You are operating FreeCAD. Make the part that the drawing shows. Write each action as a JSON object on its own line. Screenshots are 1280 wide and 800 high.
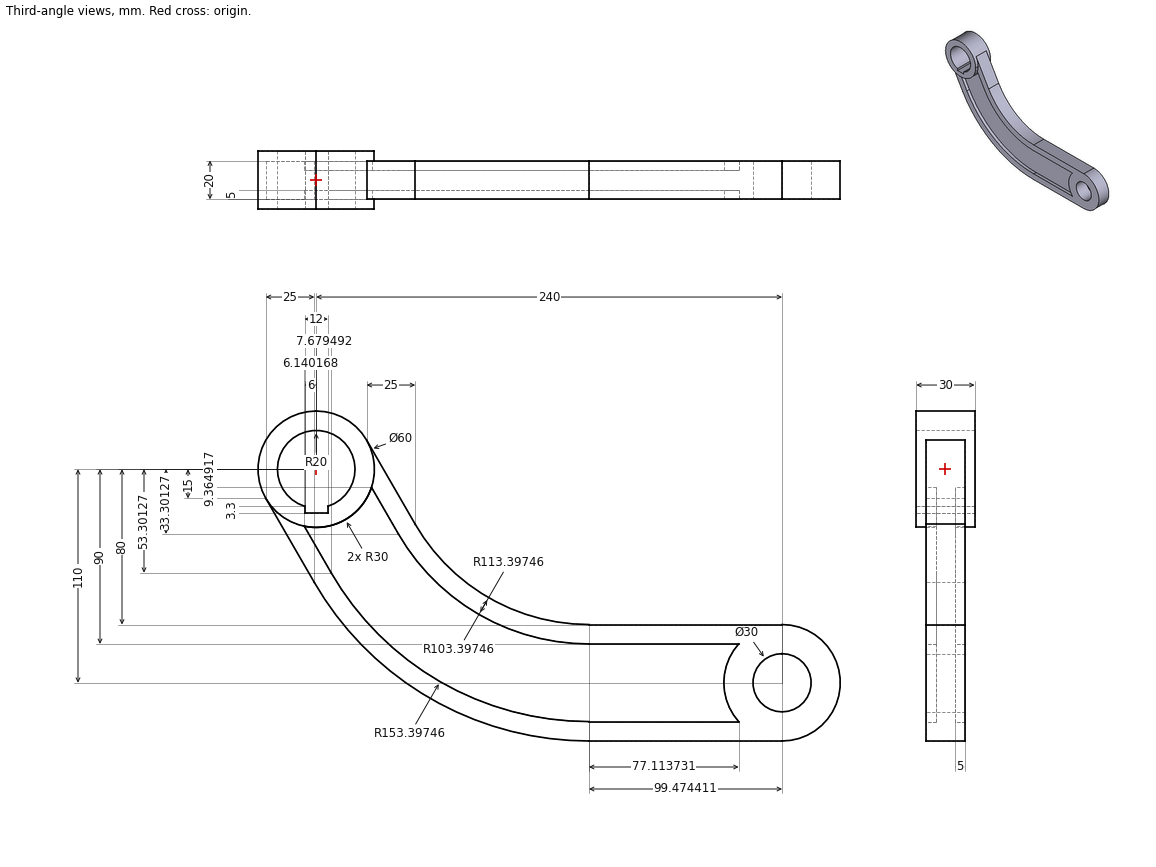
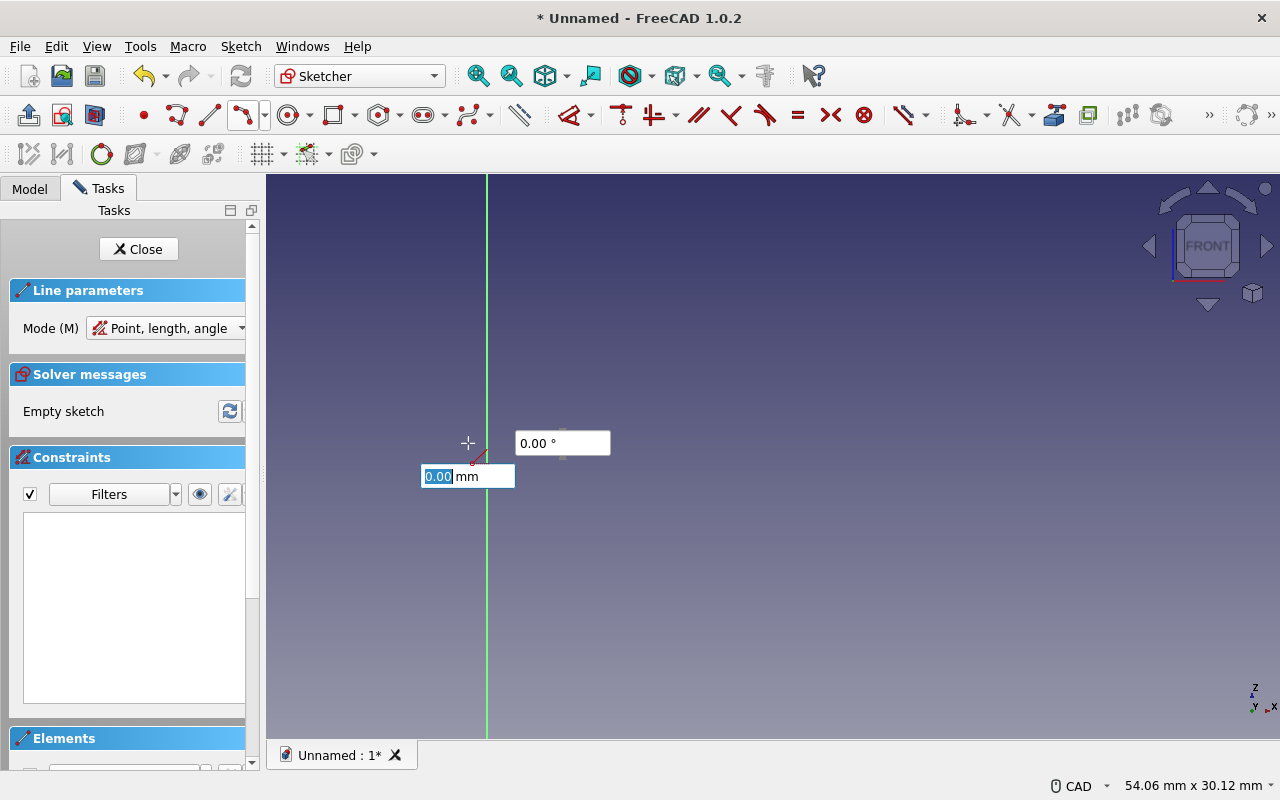
{"action": "scroll", "coordinate": [446, 448], "scroll_direction": "down", "scroll_amount": 11}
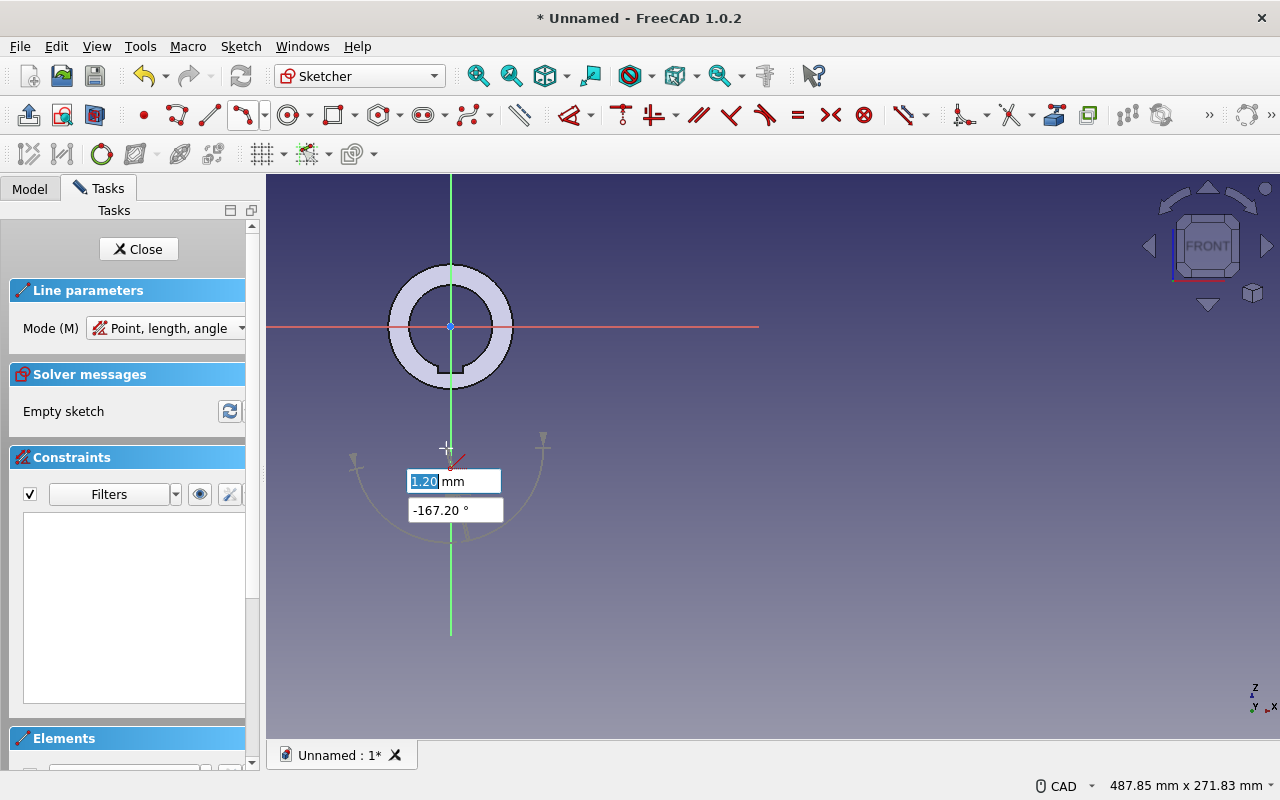
{"action": "left_click", "coordinate": [397, 358]}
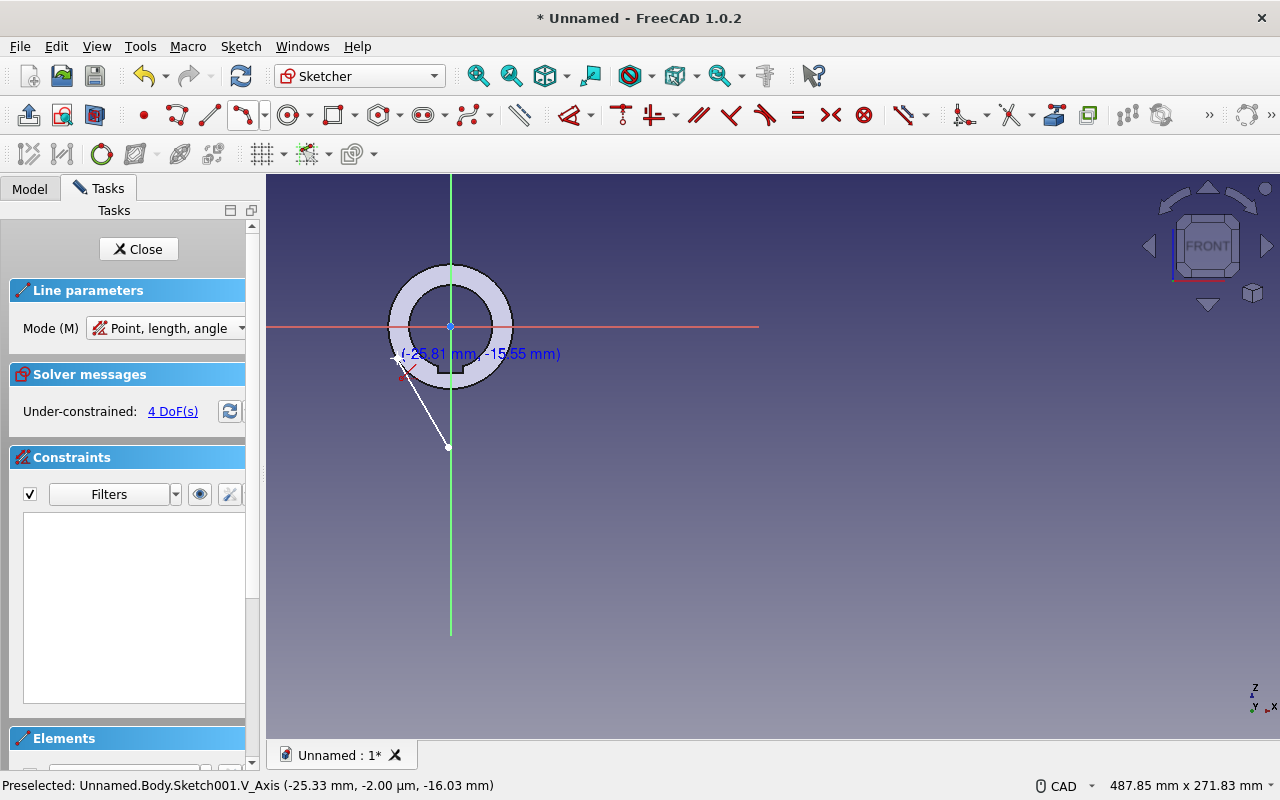
{"action": "left_click", "coordinate": [505, 296]}
{"action": "left_click", "coordinate": [557, 386]}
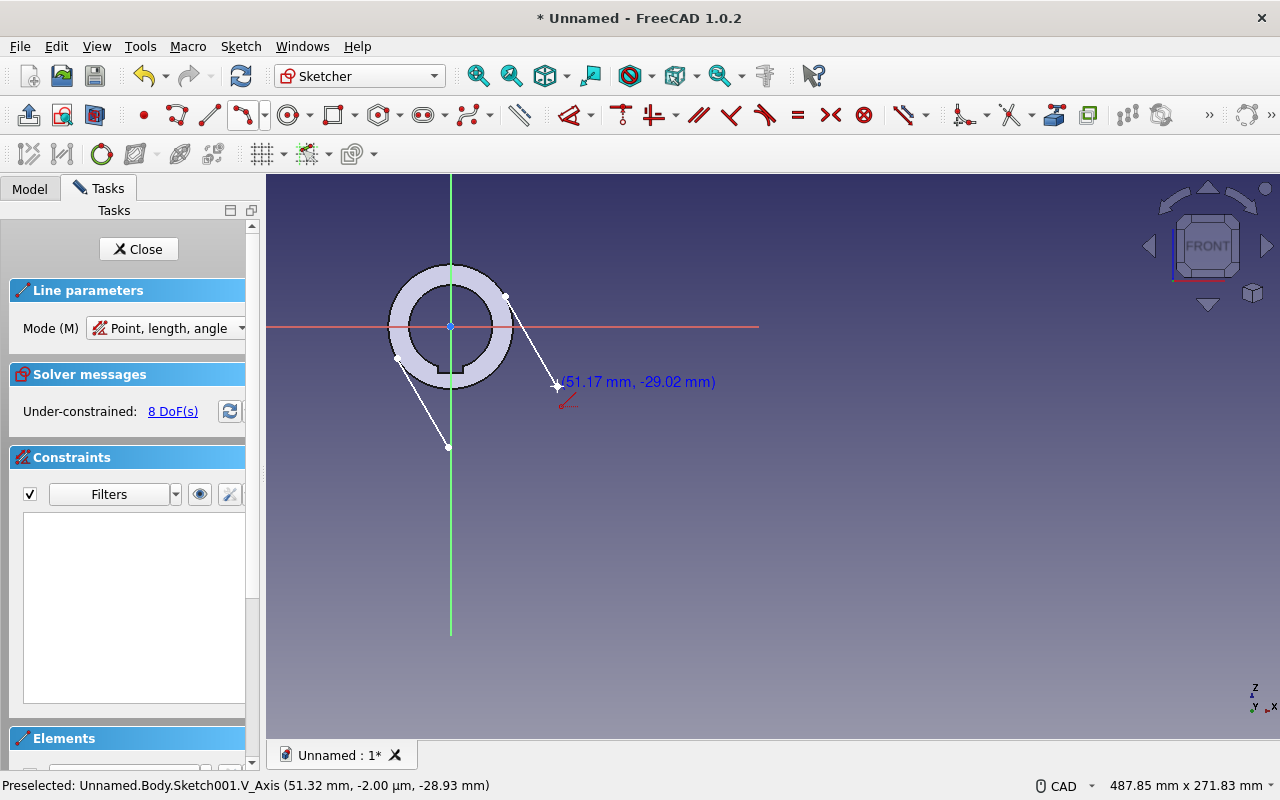
{"action": "left_click", "coordinate": [743, 493]}
{"action": "left_click", "coordinate": [949, 493]}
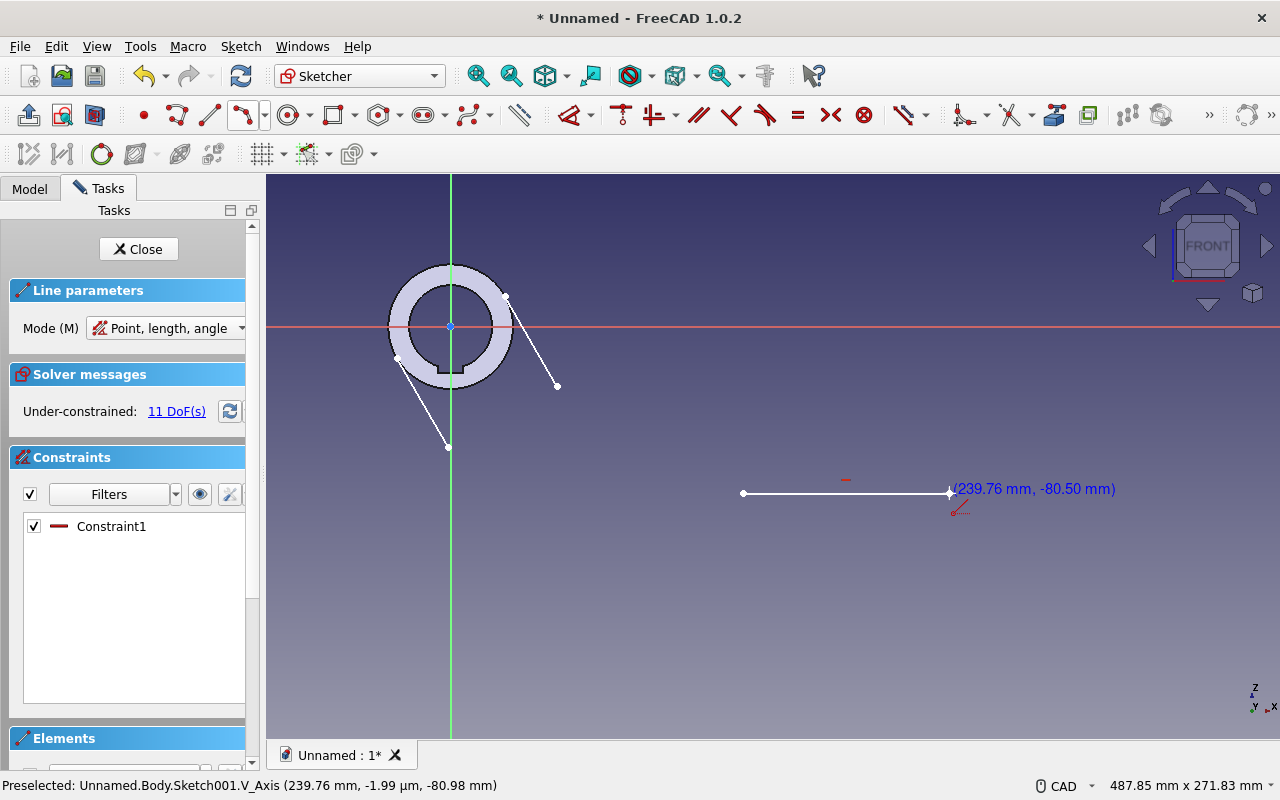
{"action": "left_click", "coordinate": [949, 618]}
{"action": "left_click", "coordinate": [743, 618]}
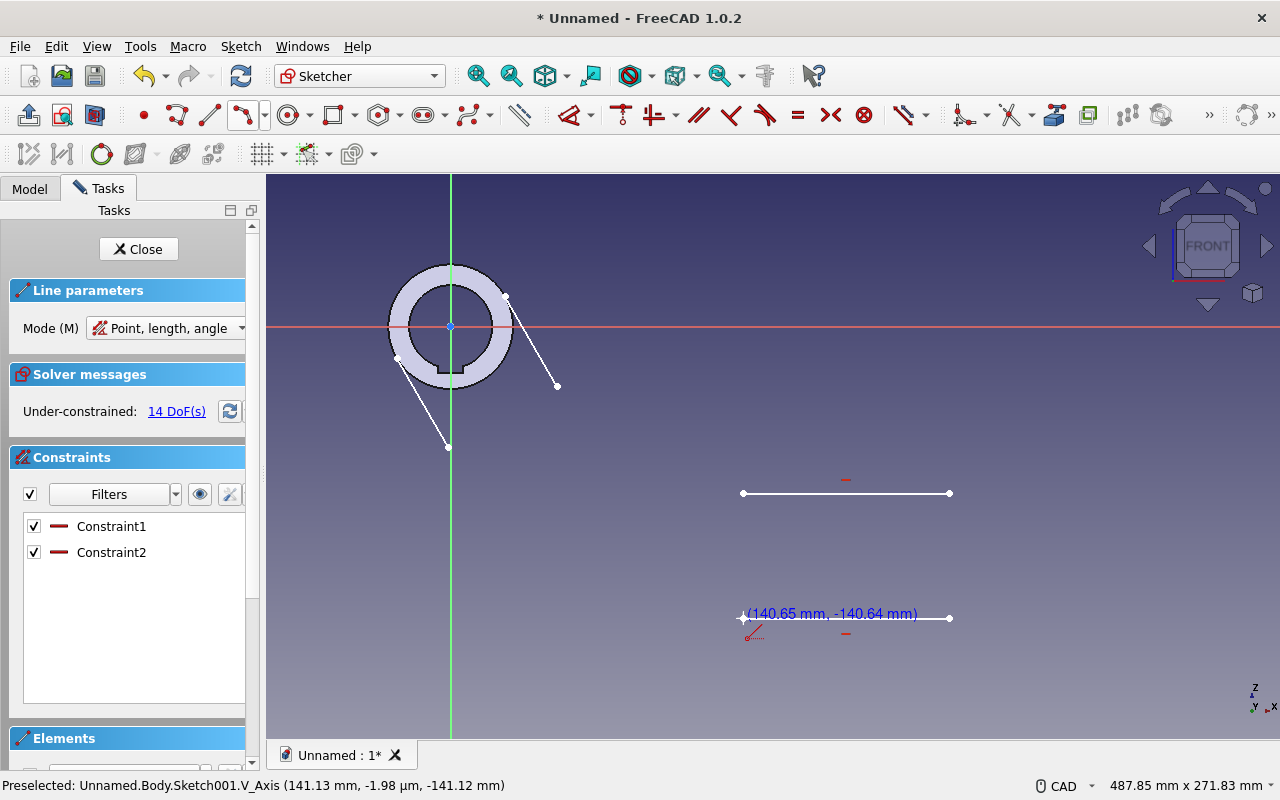
{"action": "key", "text": "g 3 a"}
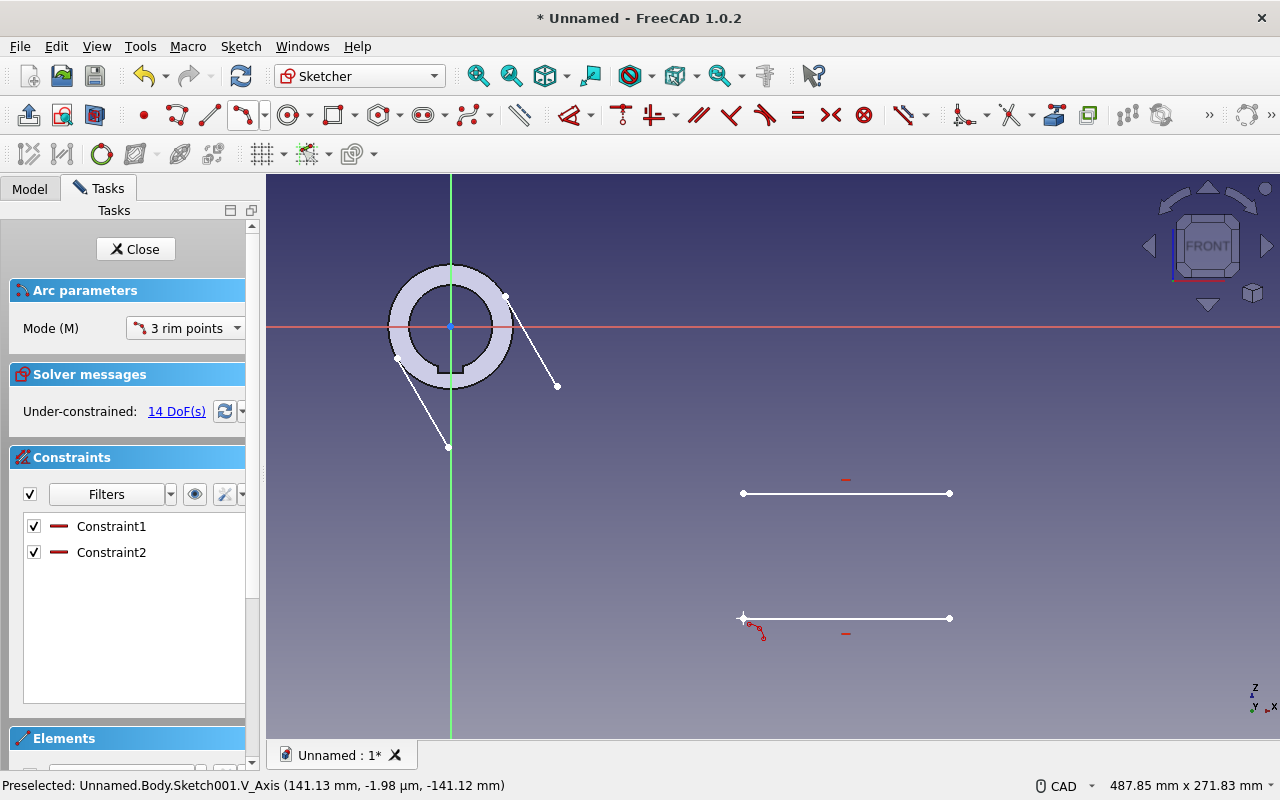
{"action": "left_click", "coordinate": [397, 359]}
{"action": "left_click", "coordinate": [505, 297]}
{"action": "left_click", "coordinate": [482, 381]}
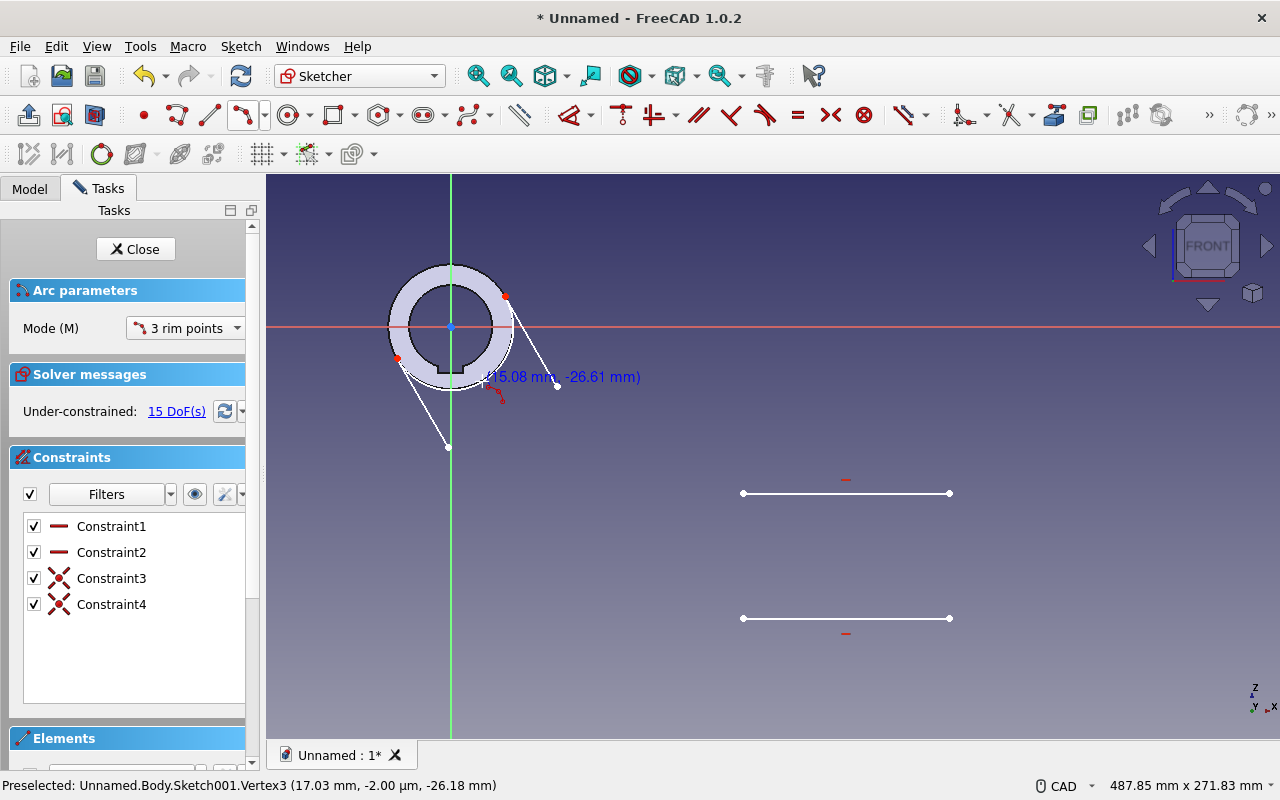
{"action": "left_click", "coordinate": [557, 387]}
{"action": "left_click", "coordinate": [743, 494]}
{"action": "left_click", "coordinate": [635, 464]}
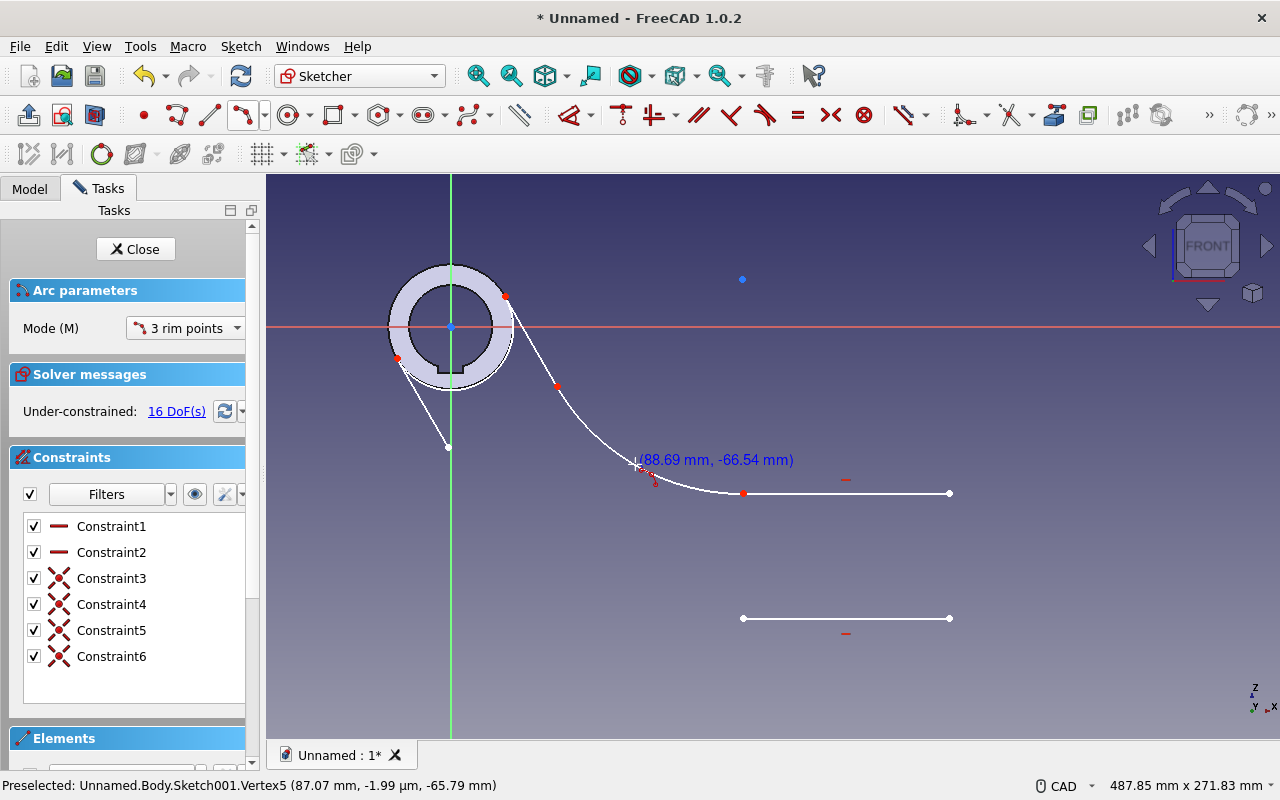
{"action": "left_click", "coordinate": [949, 494]}
{"action": "left_click", "coordinate": [949, 619]}
{"action": "left_click", "coordinate": [1012, 555]}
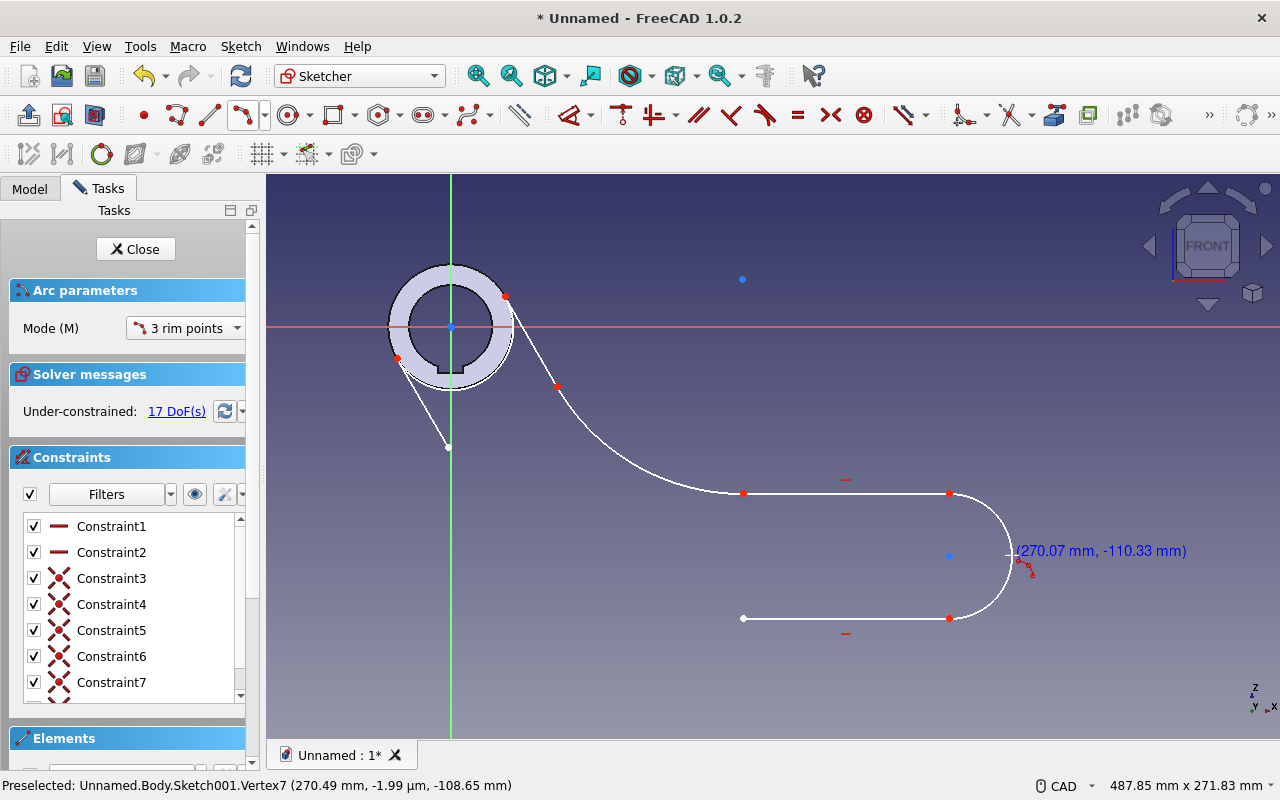
{"action": "left_click", "coordinate": [743, 619]}